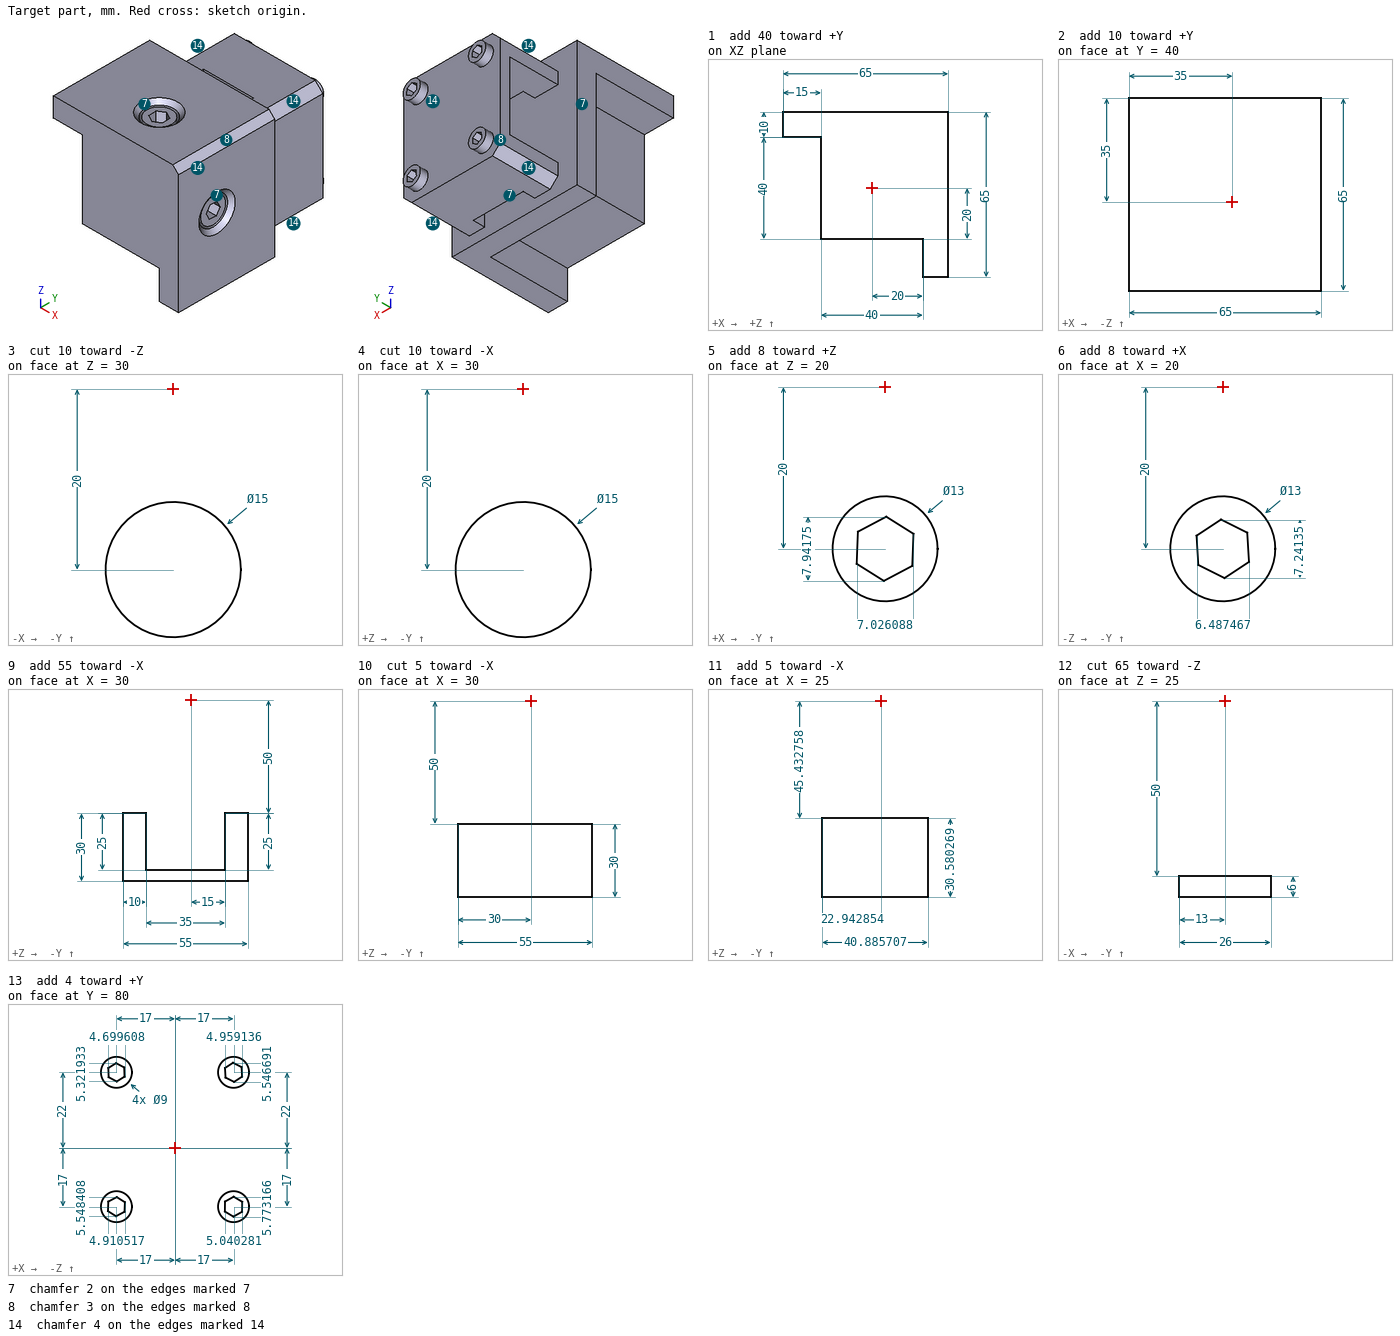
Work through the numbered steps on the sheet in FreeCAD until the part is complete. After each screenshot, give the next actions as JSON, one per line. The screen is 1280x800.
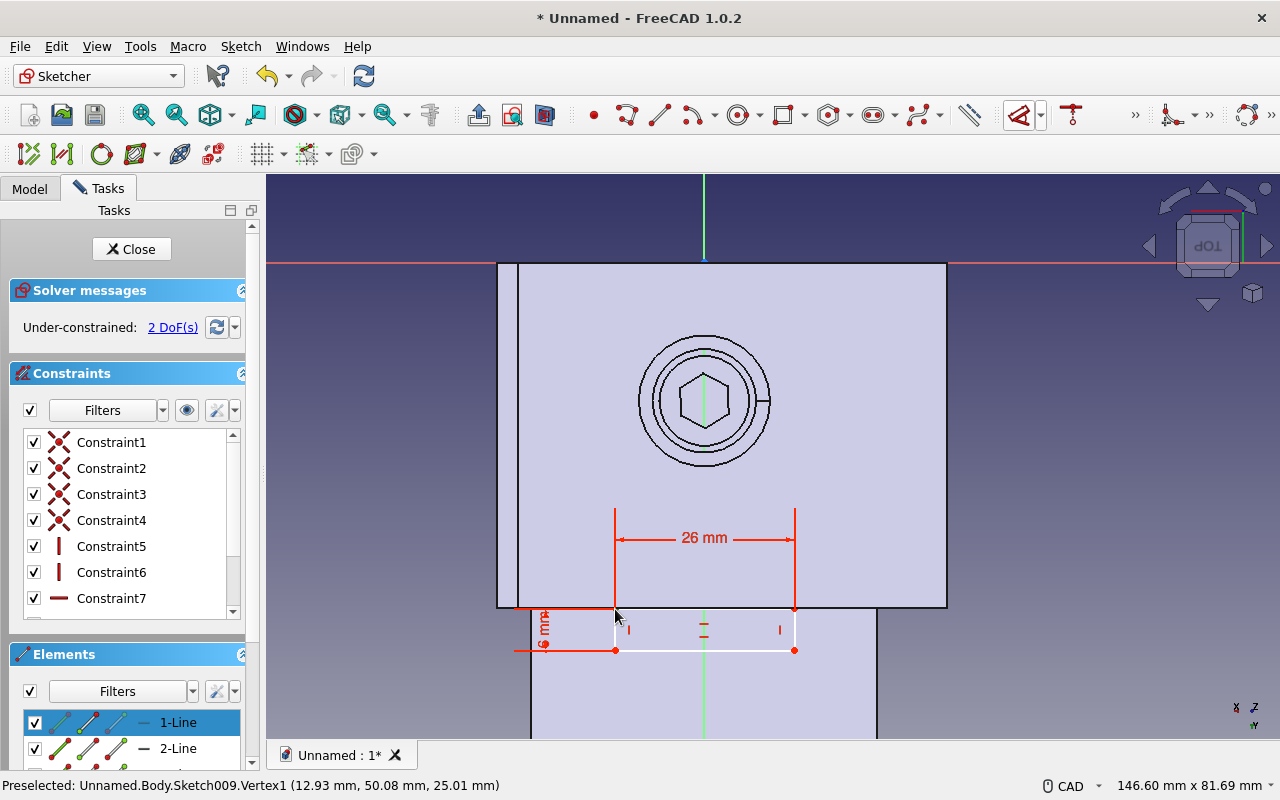
{"action": "left_click", "coordinate": [1040, 116]}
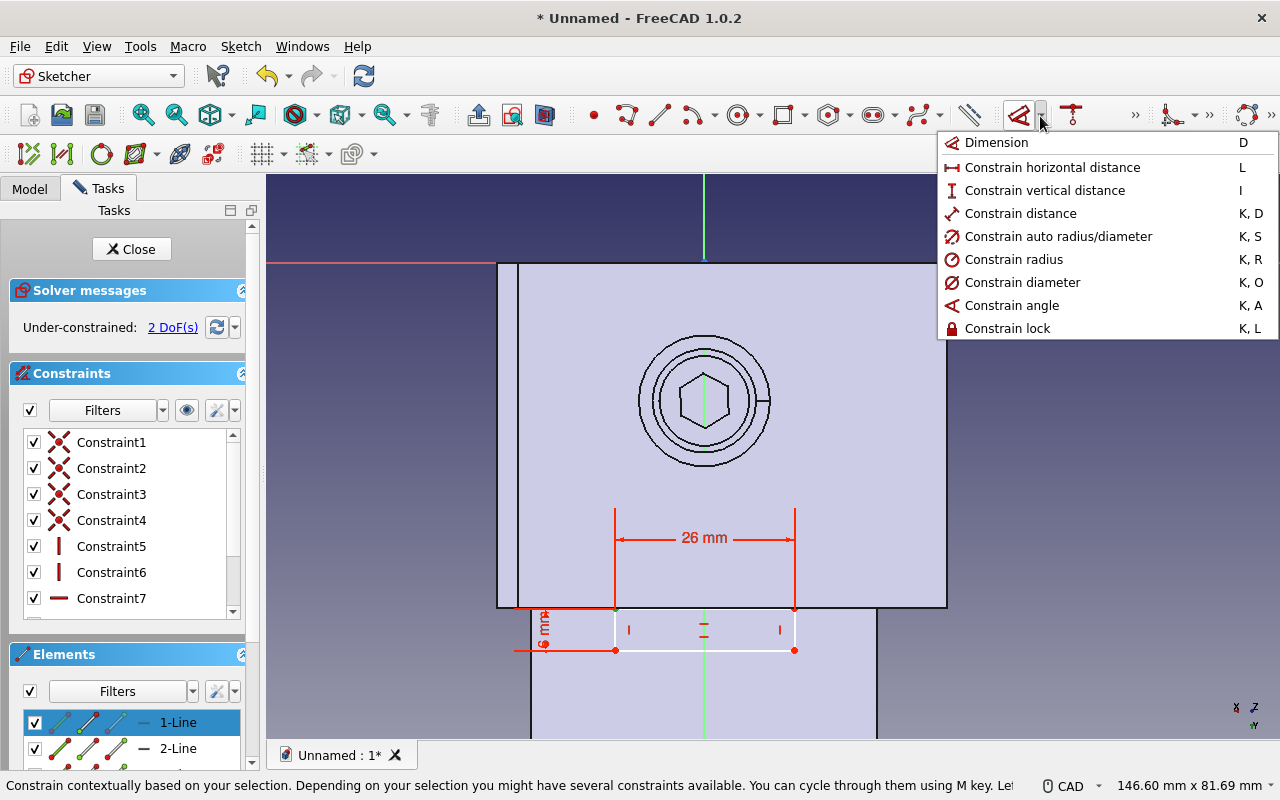
{"action": "left_click", "coordinate": [1108, 168]}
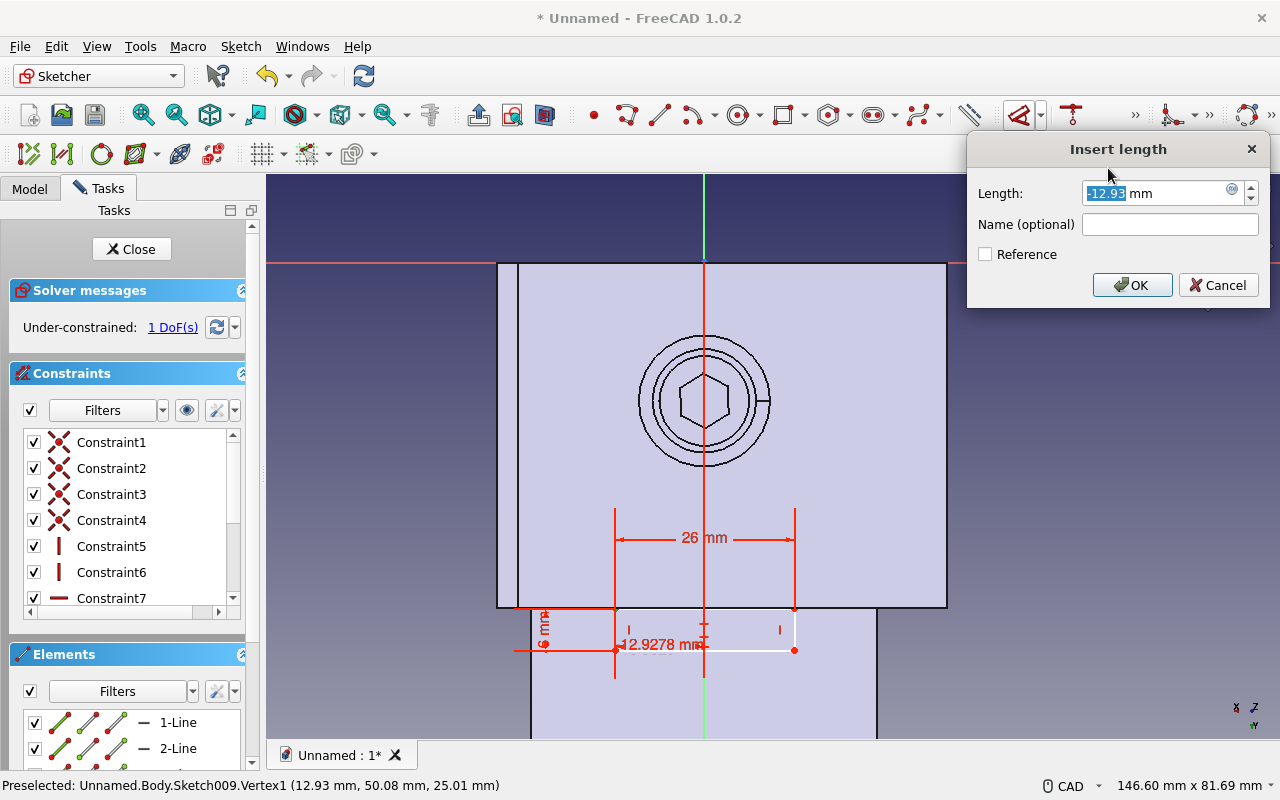
{"action": "type", "text": "-13"}
{"action": "key", "text": "Return"}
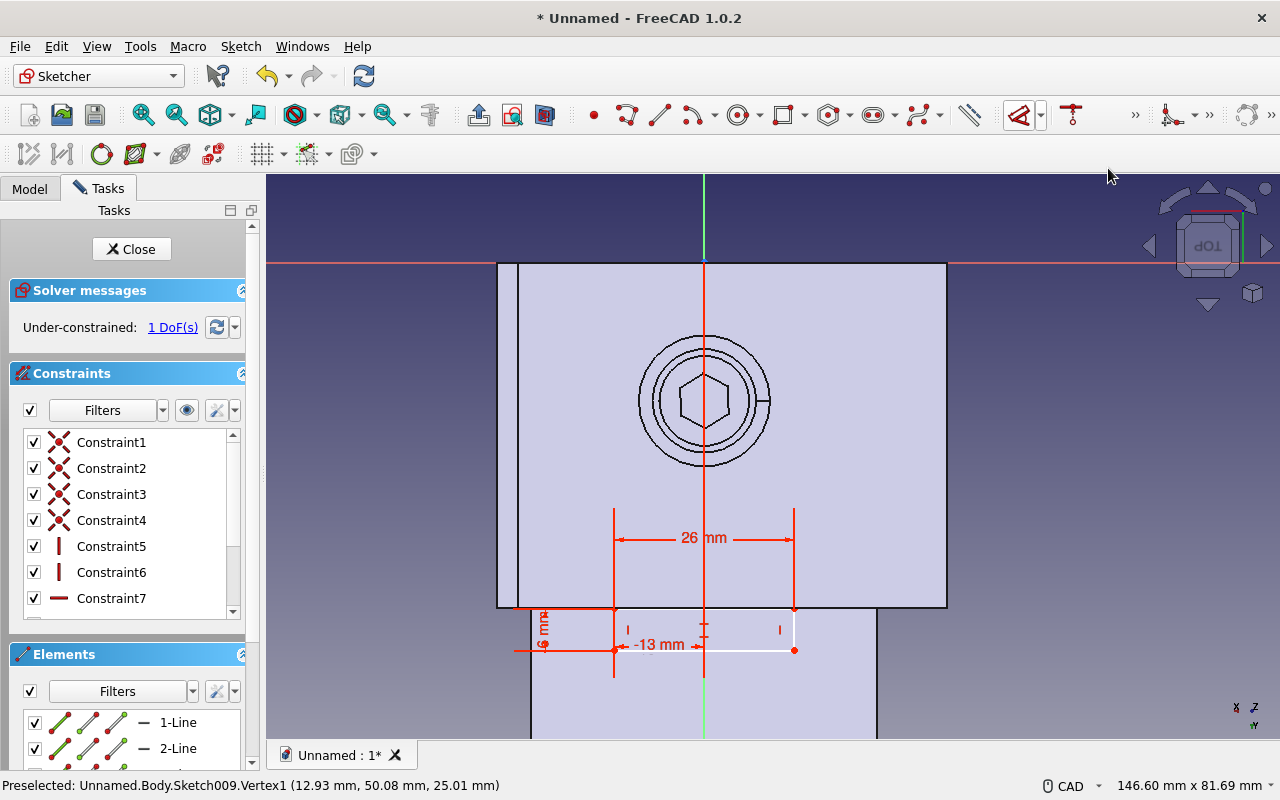
{"action": "left_click", "coordinate": [615, 609]}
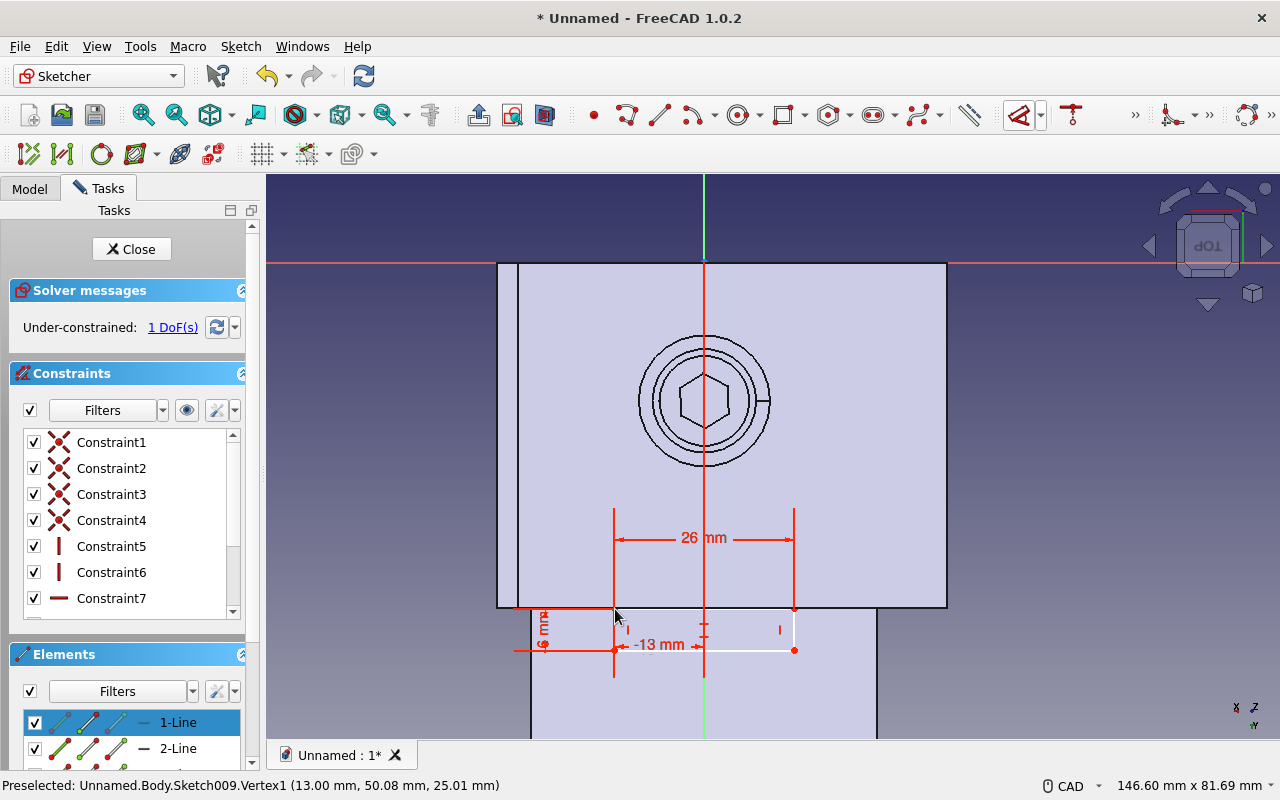
{"action": "key", "text": "i"}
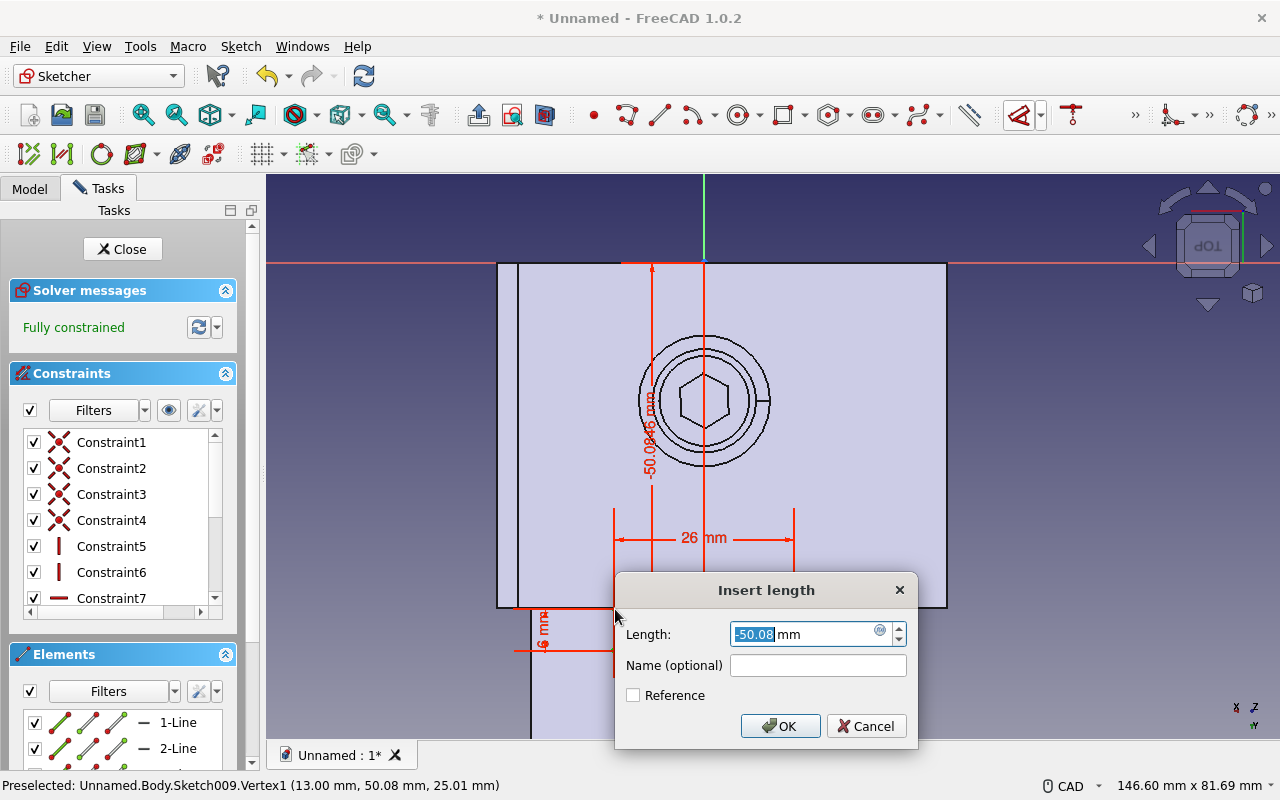
{"action": "type", "text": "-50"}
{"action": "key", "text": "Return"}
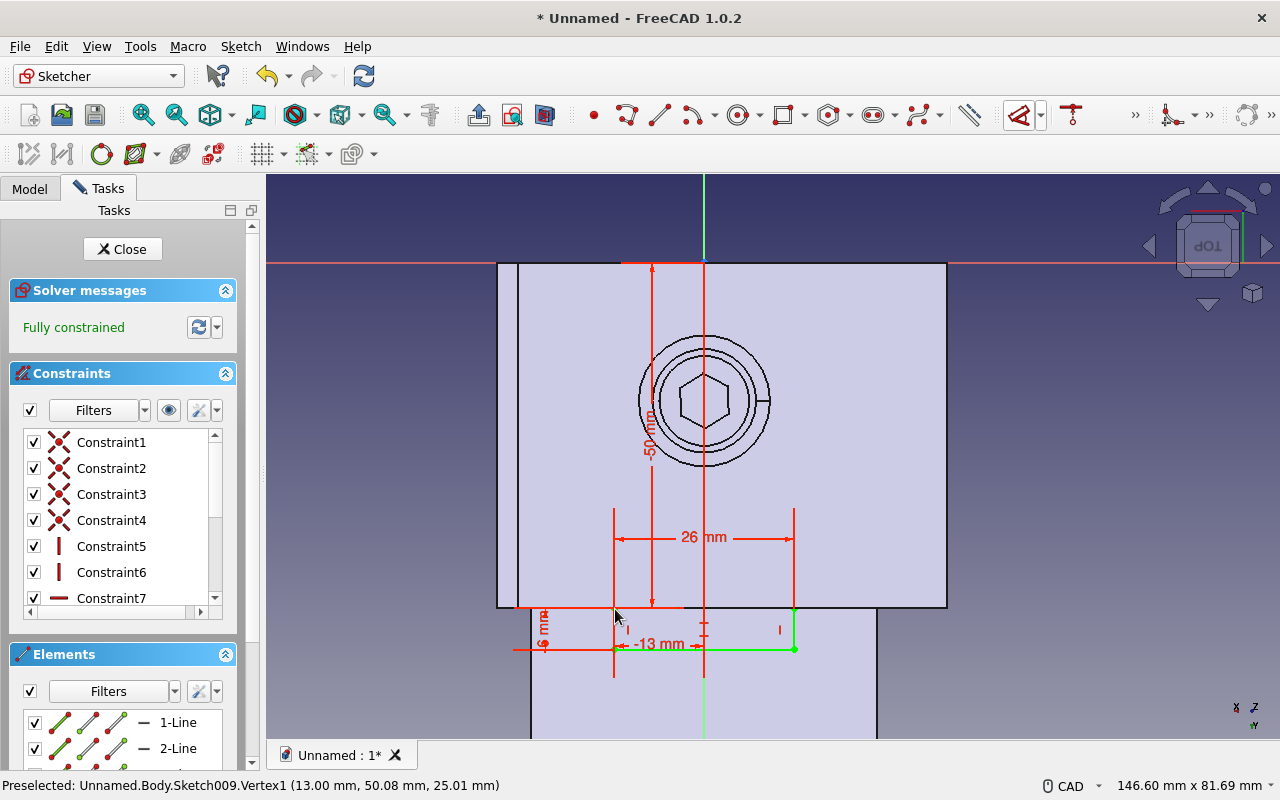
{"action": "left_click", "coordinate": [123, 249]}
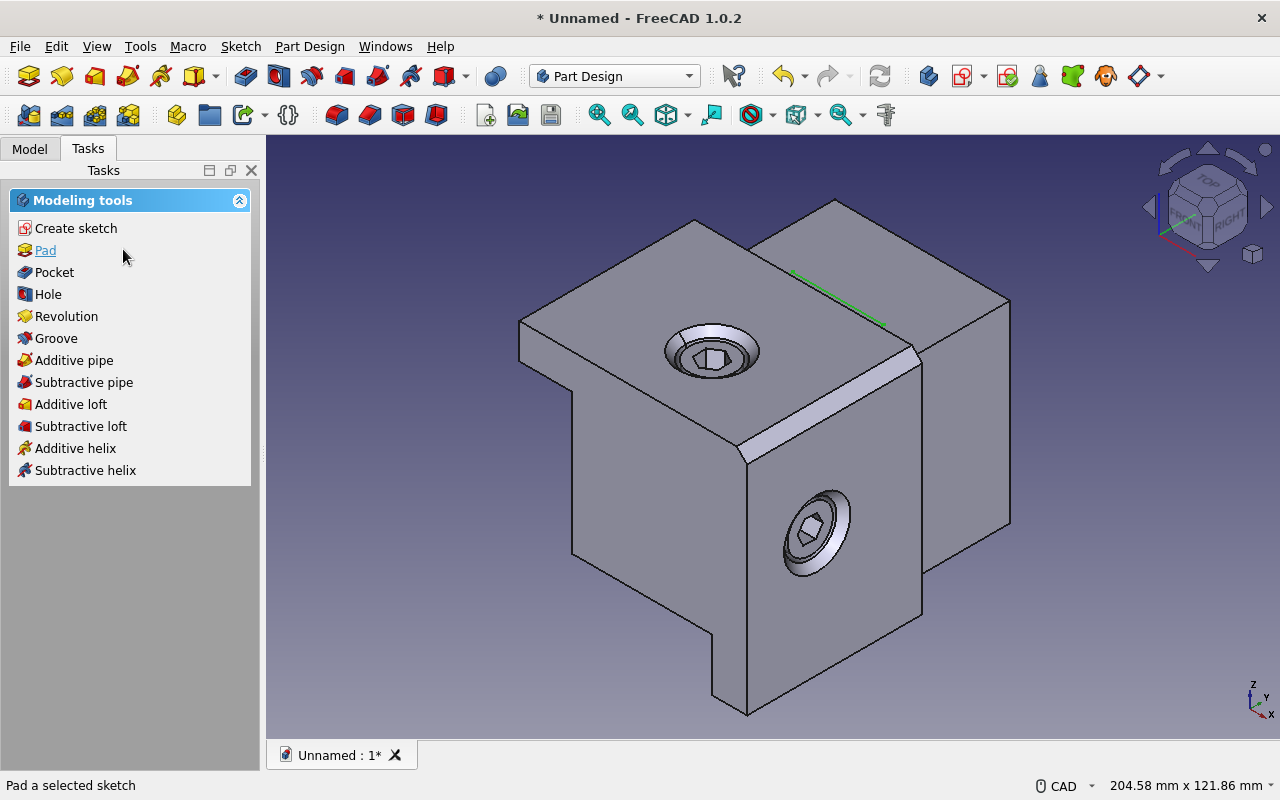
{"action": "left_click", "coordinate": [246, 76]}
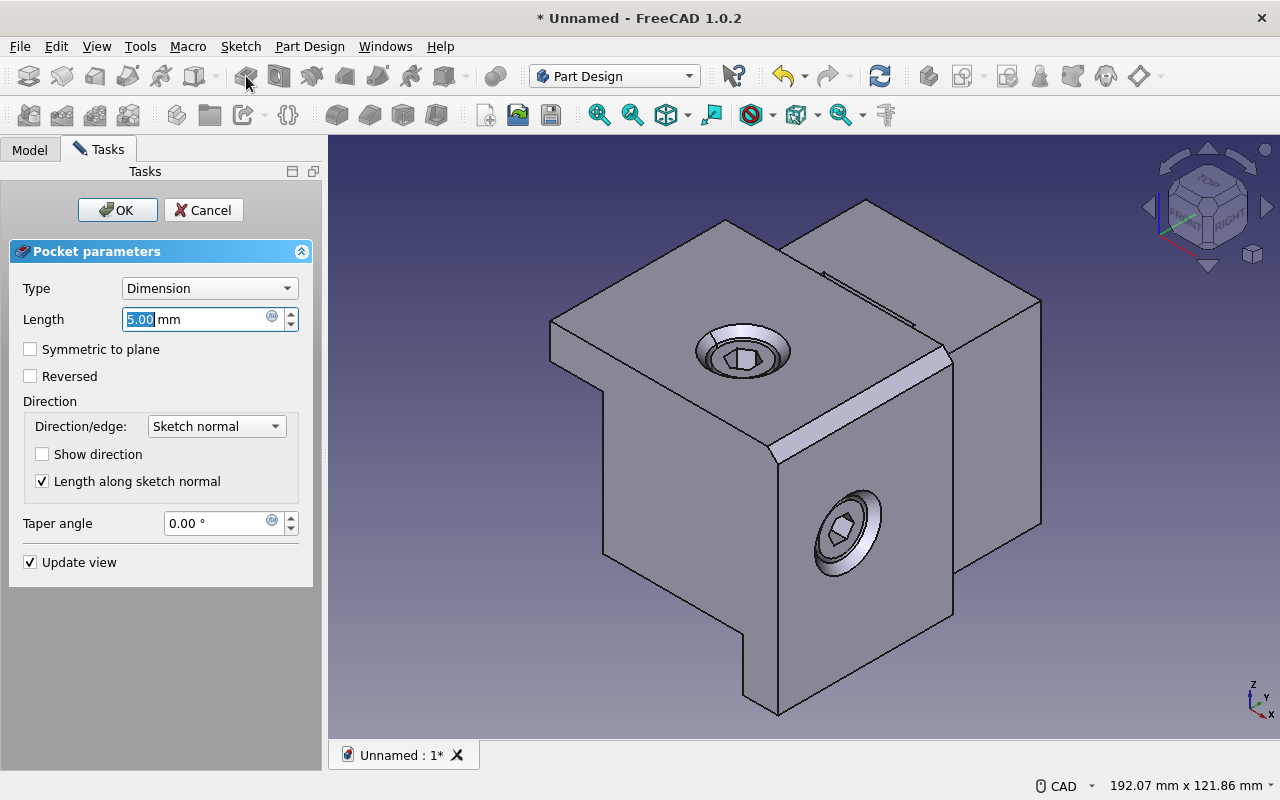
{"action": "type", "text": "65"}
{"action": "key", "text": "Tab"}